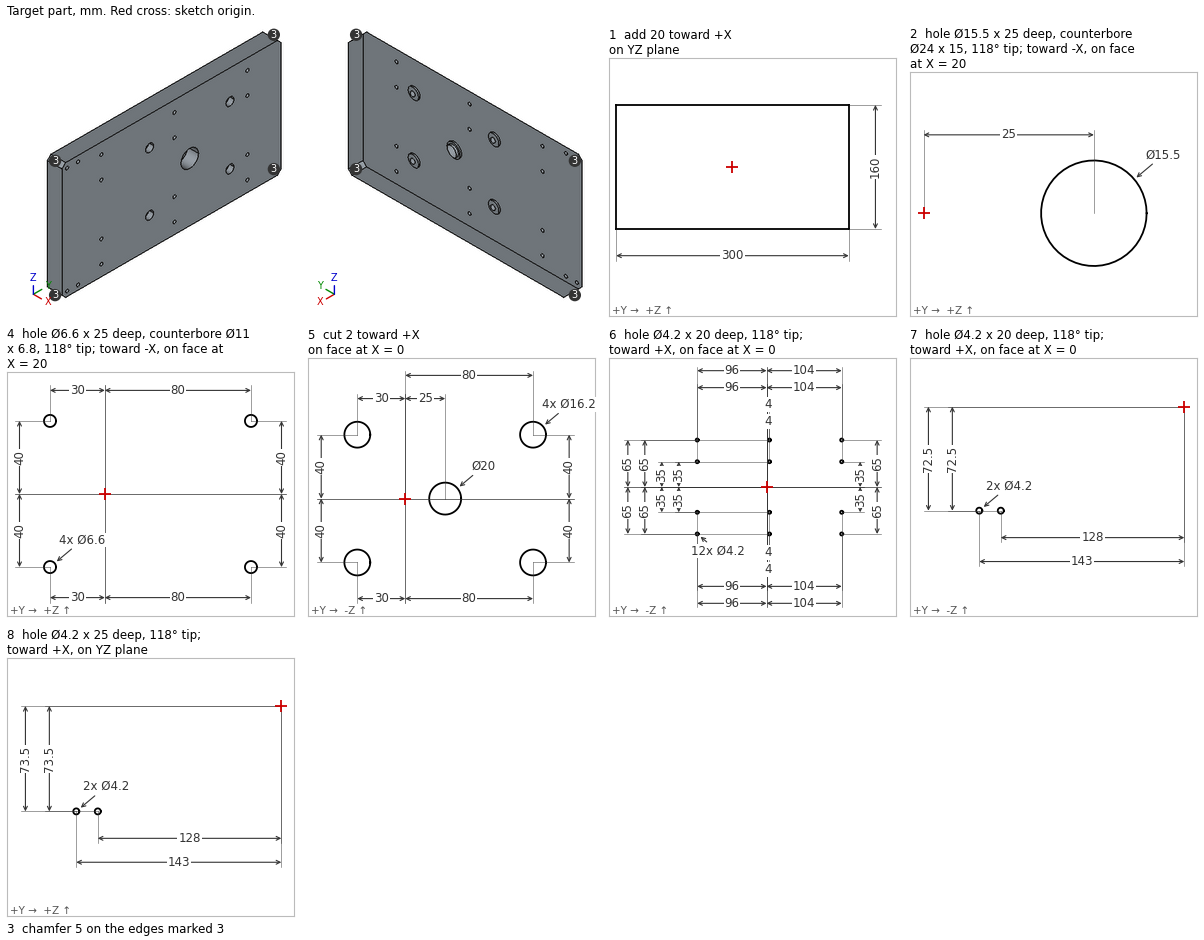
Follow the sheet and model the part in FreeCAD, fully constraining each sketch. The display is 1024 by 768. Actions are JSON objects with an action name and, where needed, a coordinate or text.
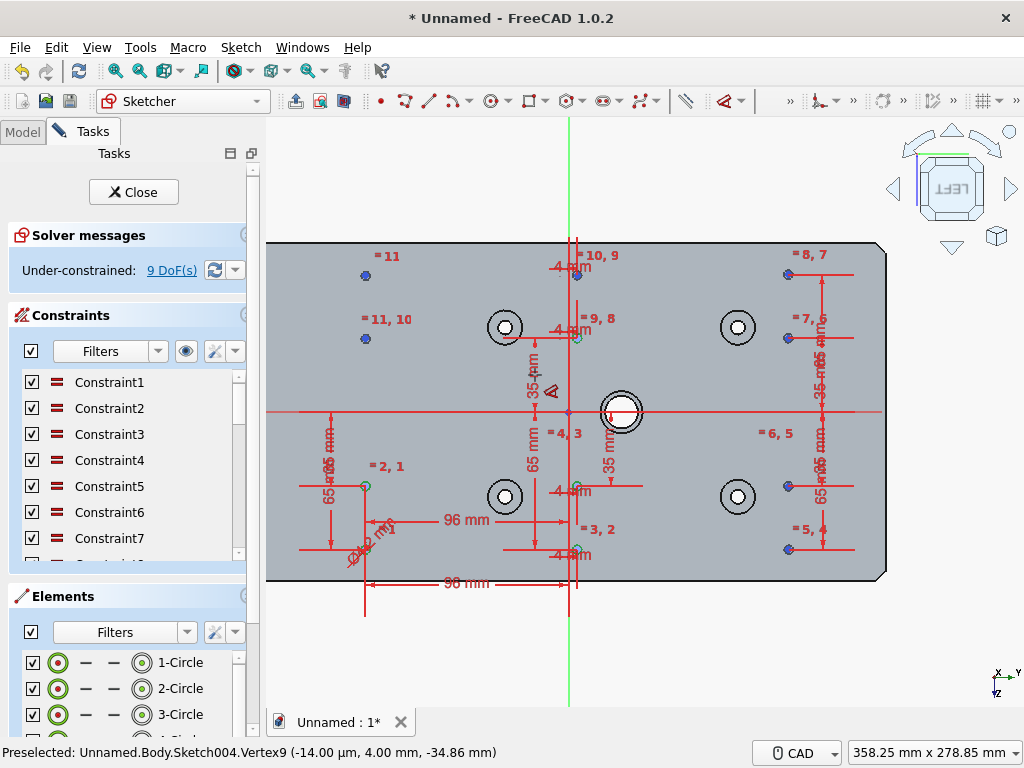
{"action": "left_click", "coordinate": [577, 275]}
{"action": "left_click", "coordinate": [535, 296]}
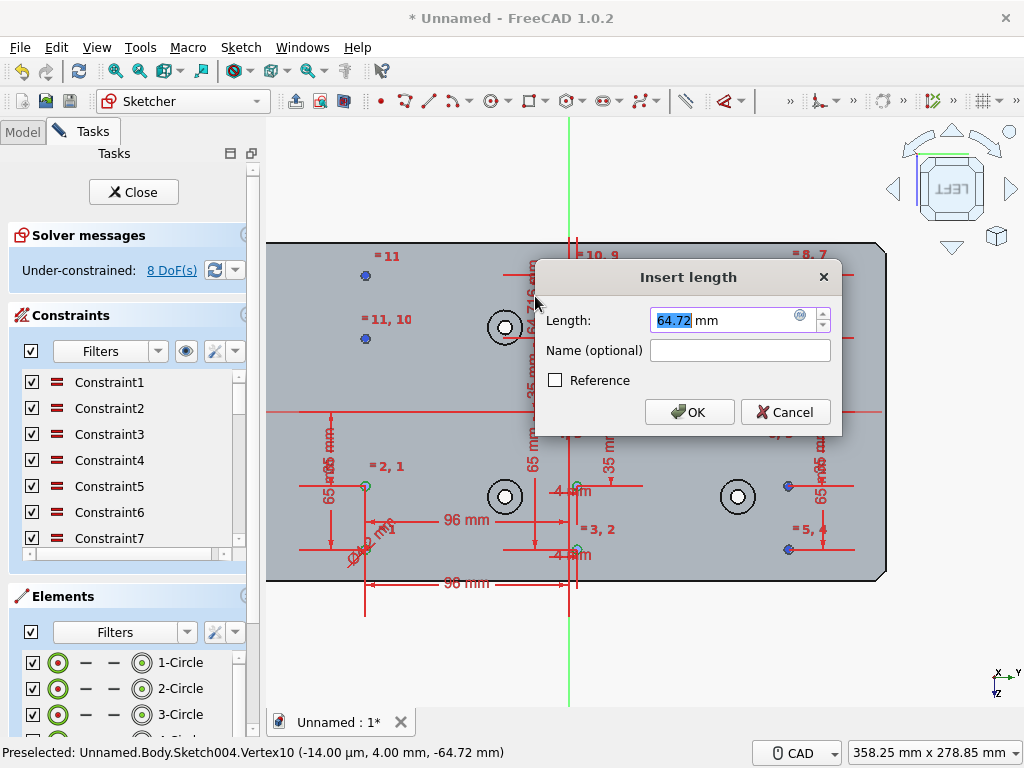
{"action": "type", "text": "65"}
{"action": "key", "text": "Return"}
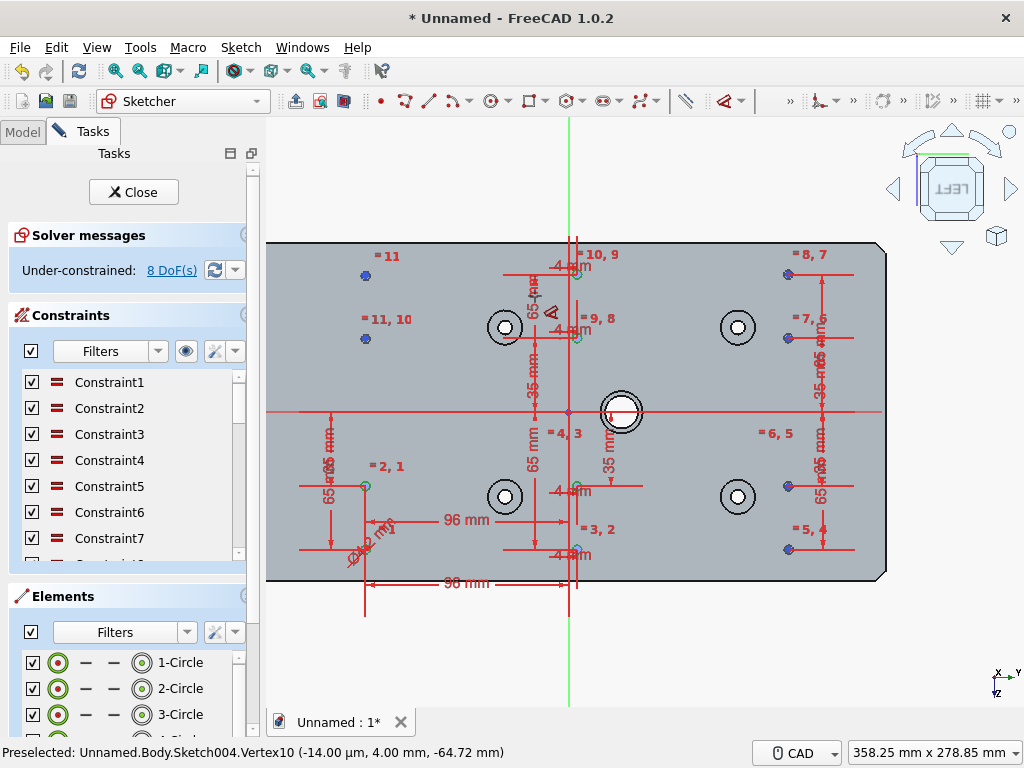
{"action": "left_click", "coordinate": [366, 339]}
{"action": "left_click", "coordinate": [421, 305]}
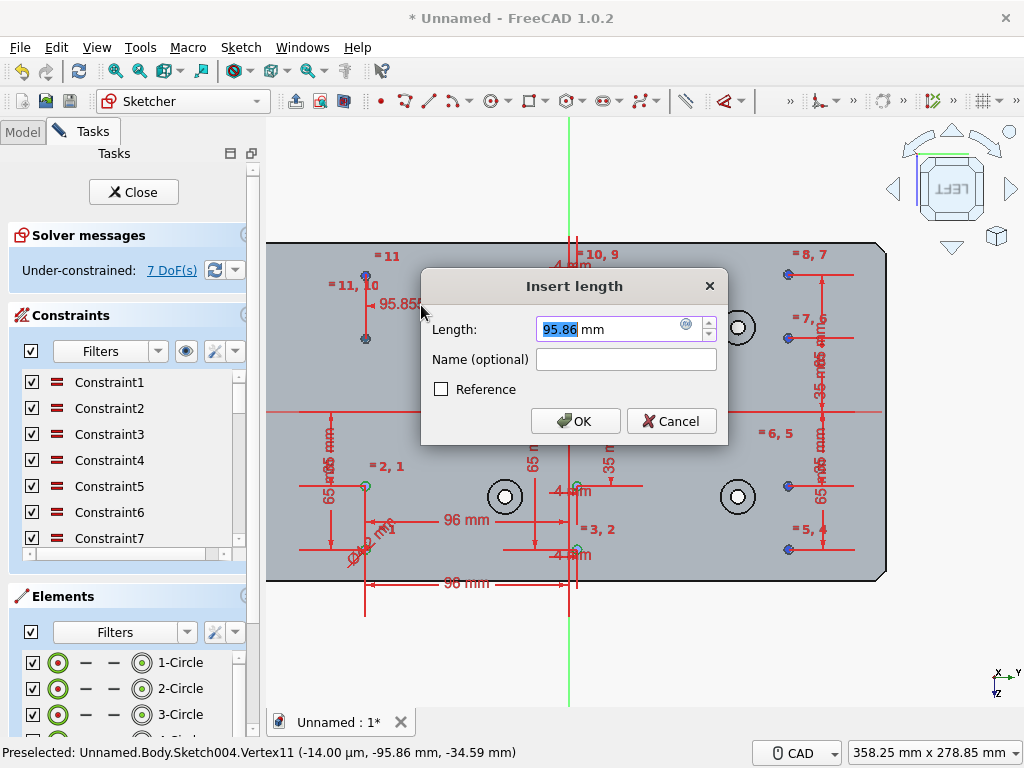
{"action": "type", "text": "96"}
{"action": "key", "text": "Return"}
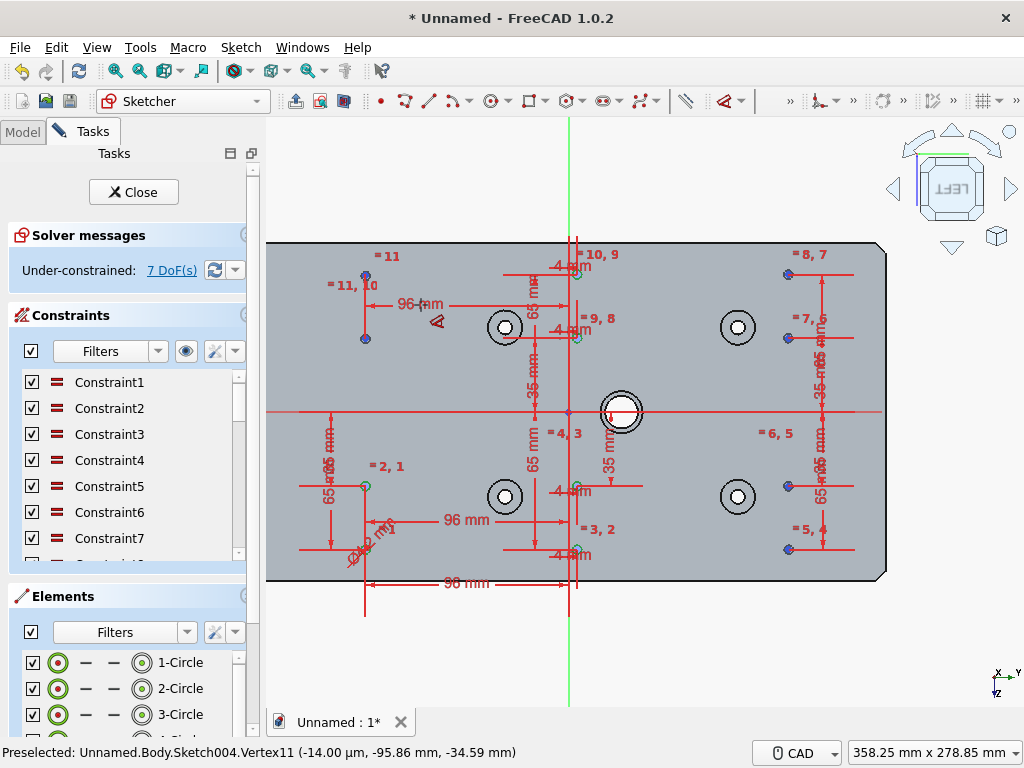
{"action": "left_click", "coordinate": [365, 339]}
{"action": "left_click", "coordinate": [331, 376]}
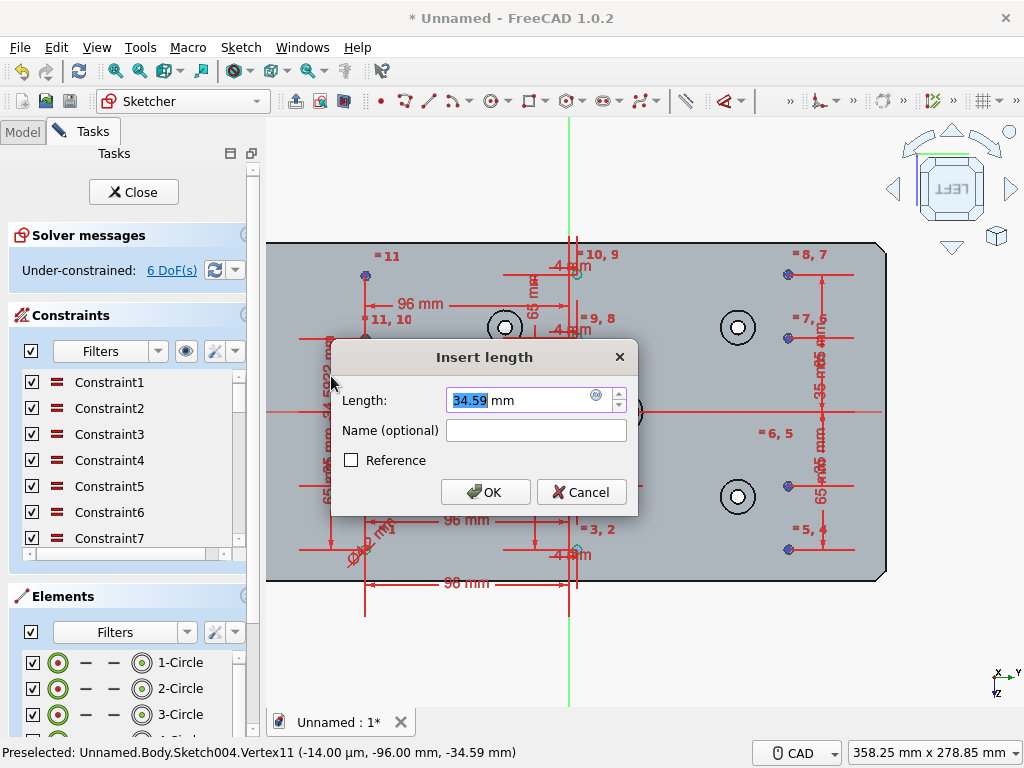
{"action": "type", "text": "35"}
{"action": "key", "text": "Return"}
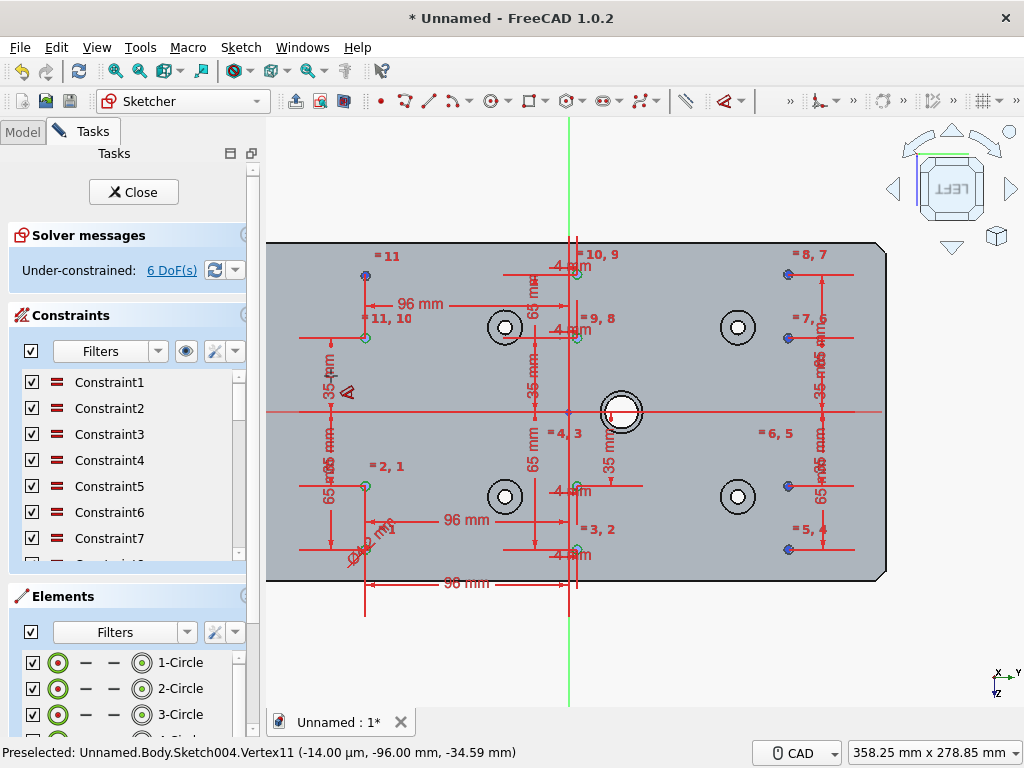
{"action": "left_click", "coordinate": [366, 276]}
{"action": "left_click", "coordinate": [467, 242]}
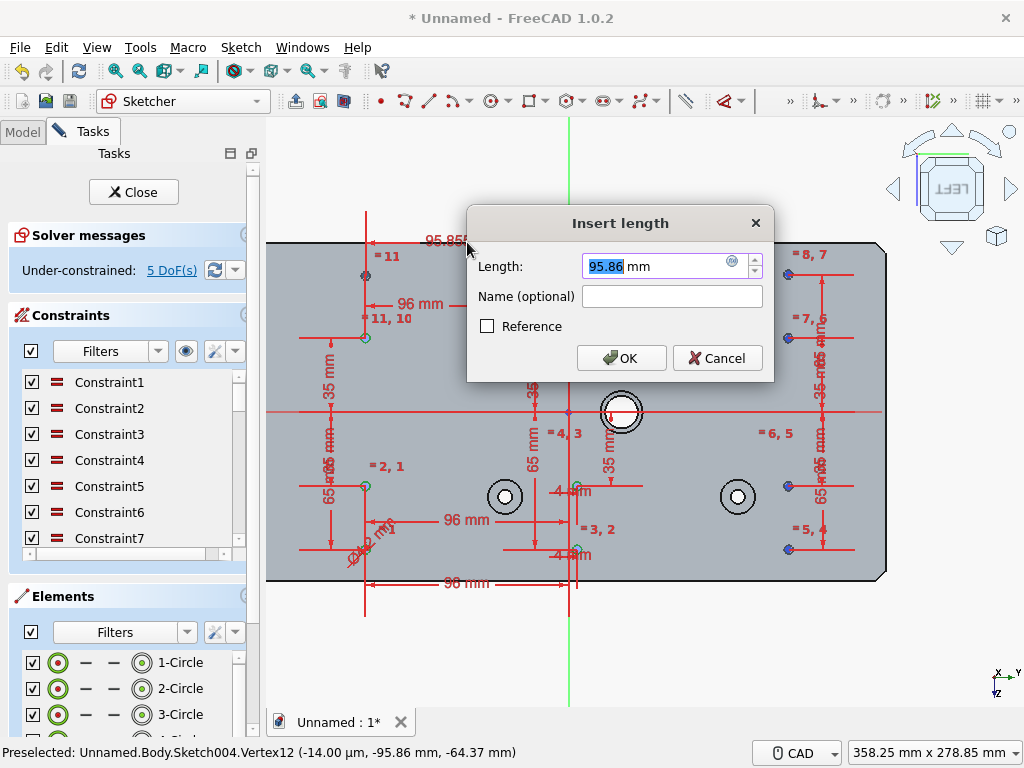
{"action": "type", "text": "96"}
{"action": "key", "text": "Return"}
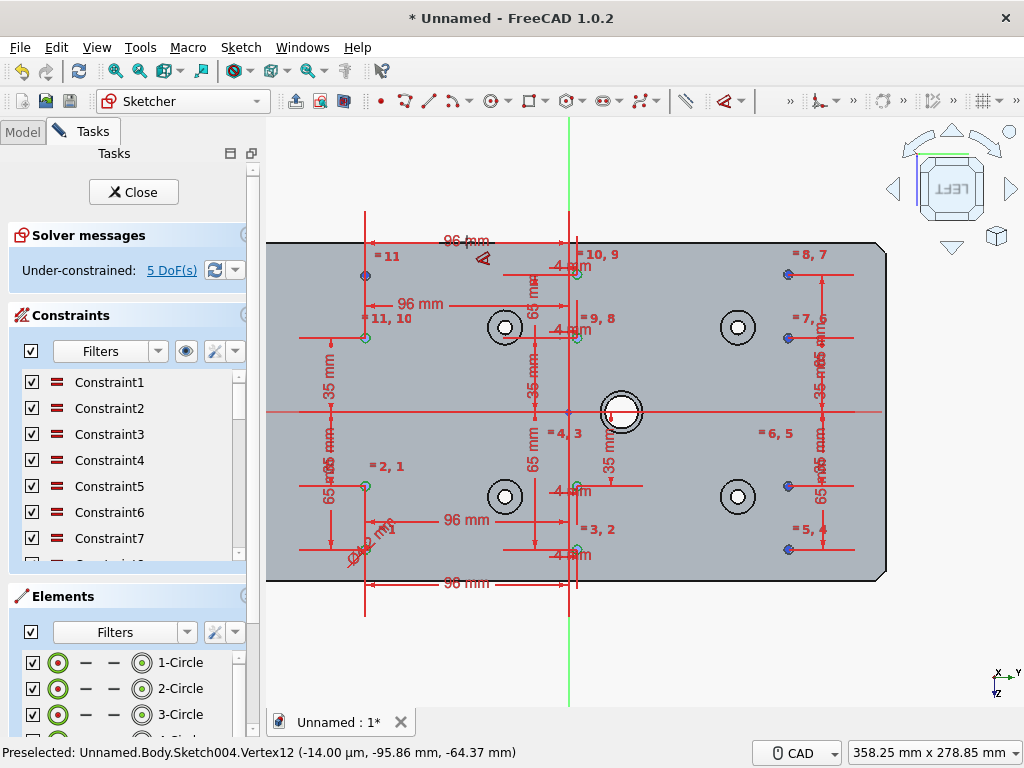
{"action": "left_click", "coordinate": [365, 276]}
{"action": "left_click", "coordinate": [331, 344]}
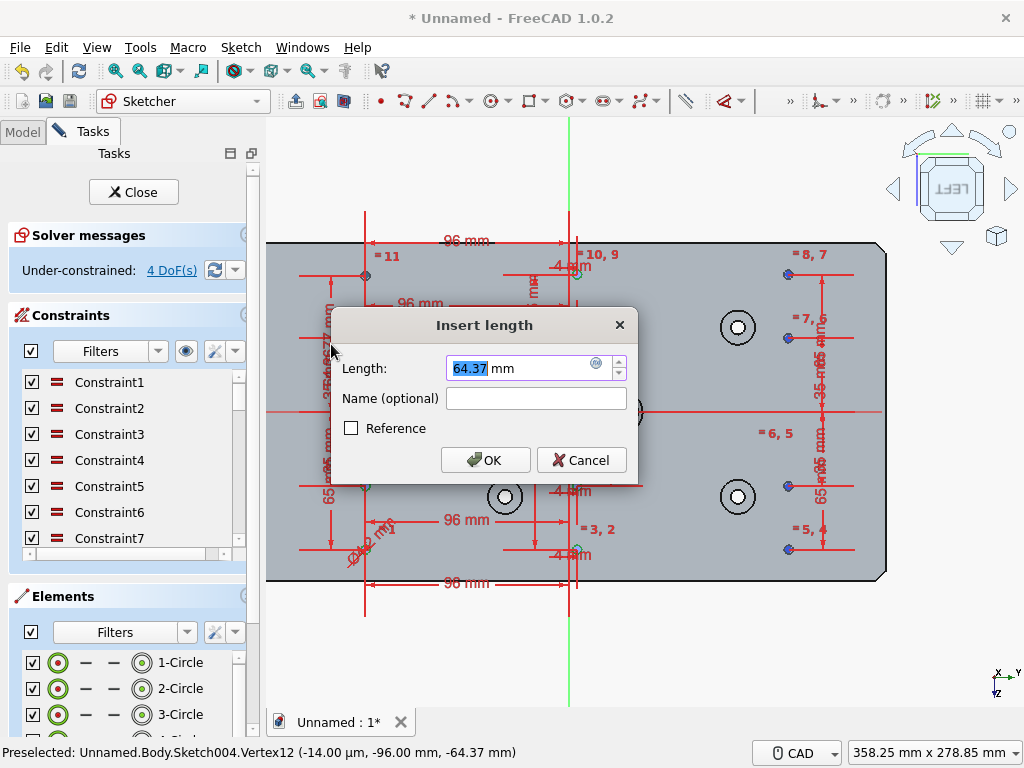
{"action": "type", "text": "65"}
{"action": "key", "text": "Return"}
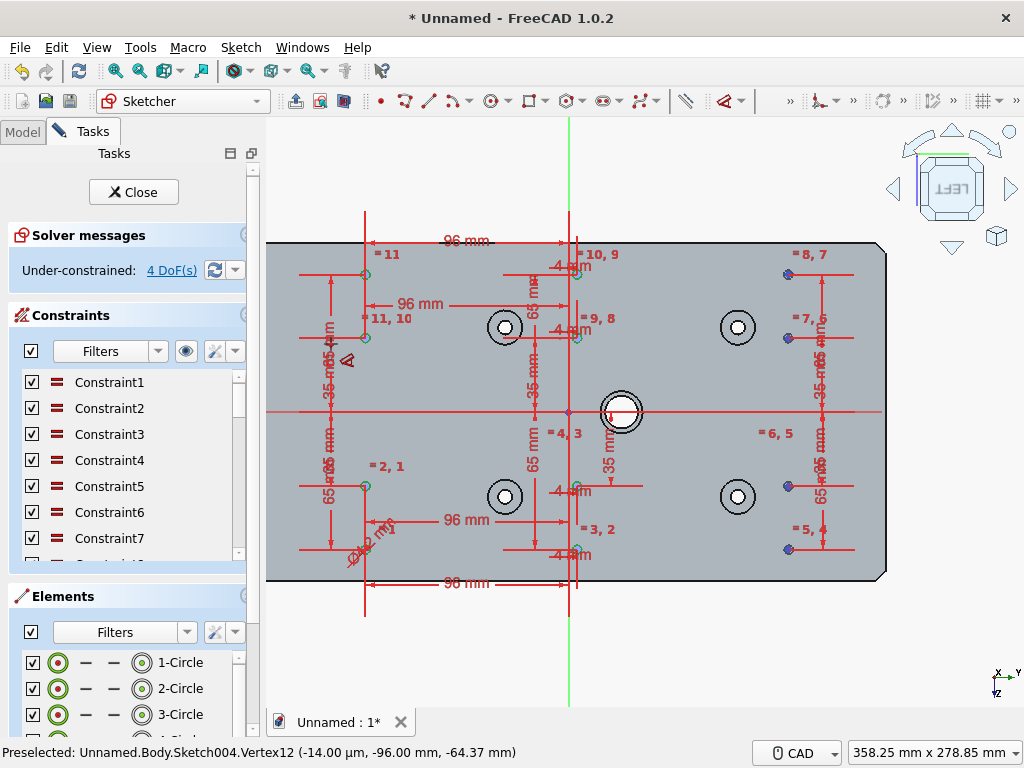
{"action": "left_click", "coordinate": [789, 550]}
{"action": "left_click", "coordinate": [679, 584]}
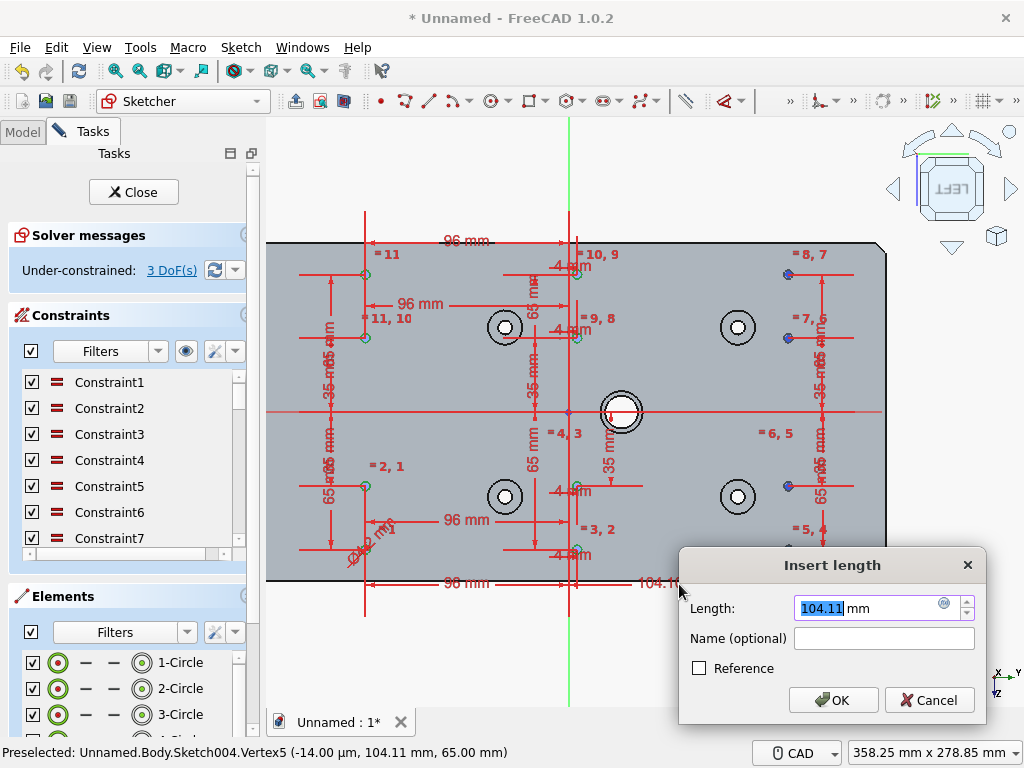
{"action": "type", "text": "104"}
{"action": "key", "text": "Return"}